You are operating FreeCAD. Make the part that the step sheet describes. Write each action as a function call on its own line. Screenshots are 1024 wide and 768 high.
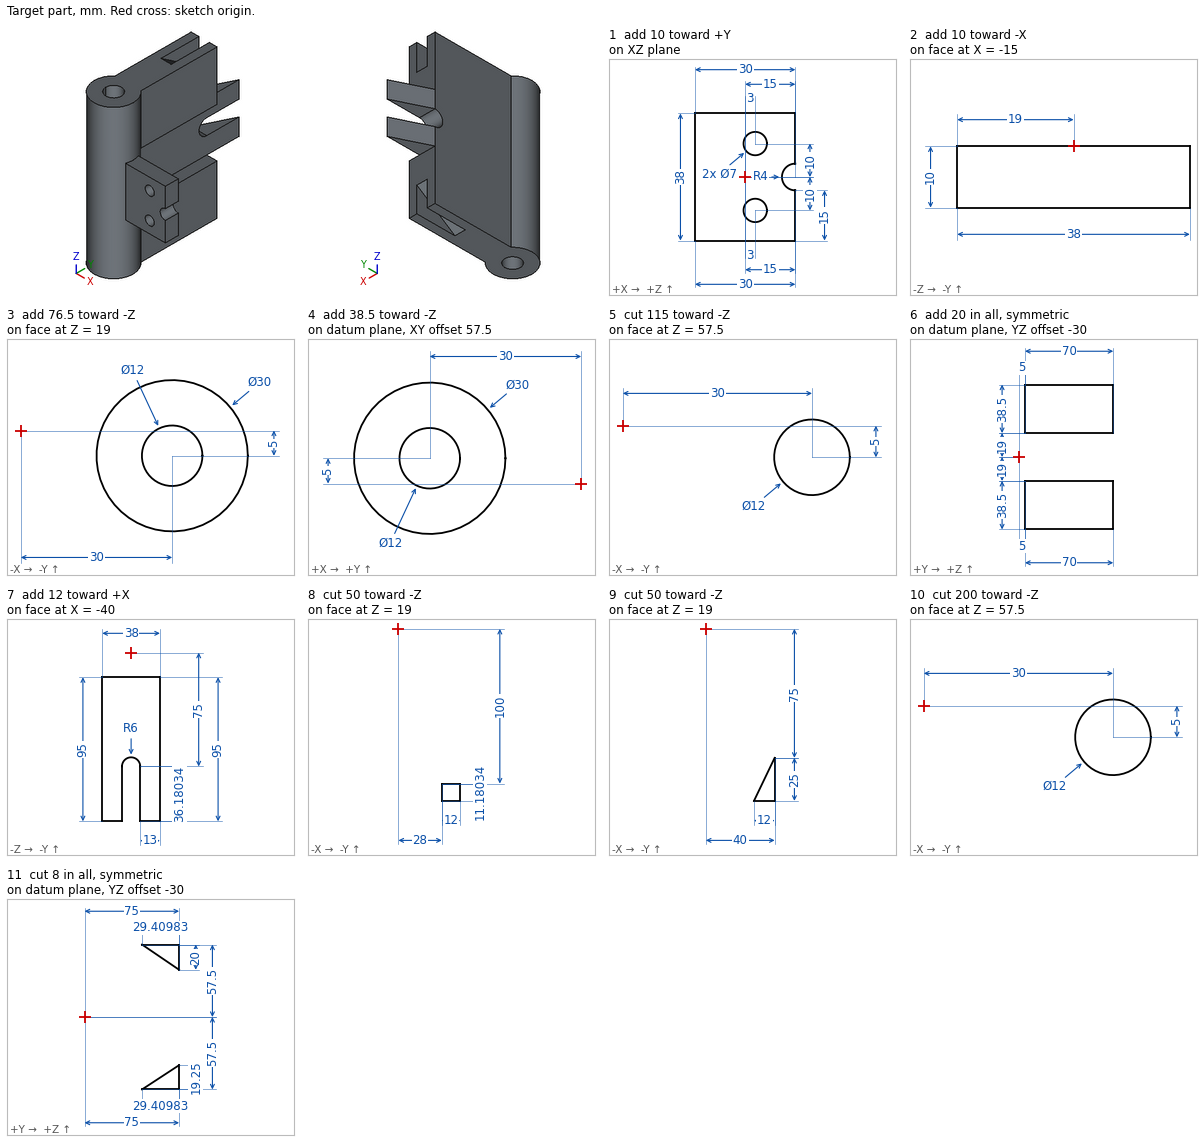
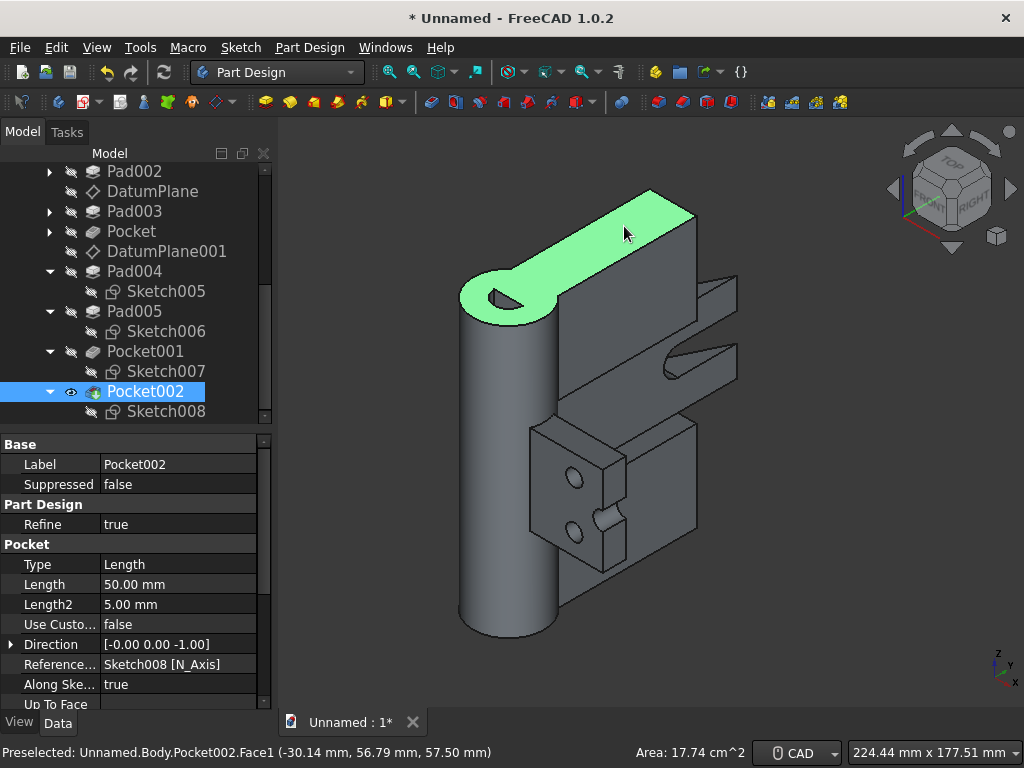
click(84, 102)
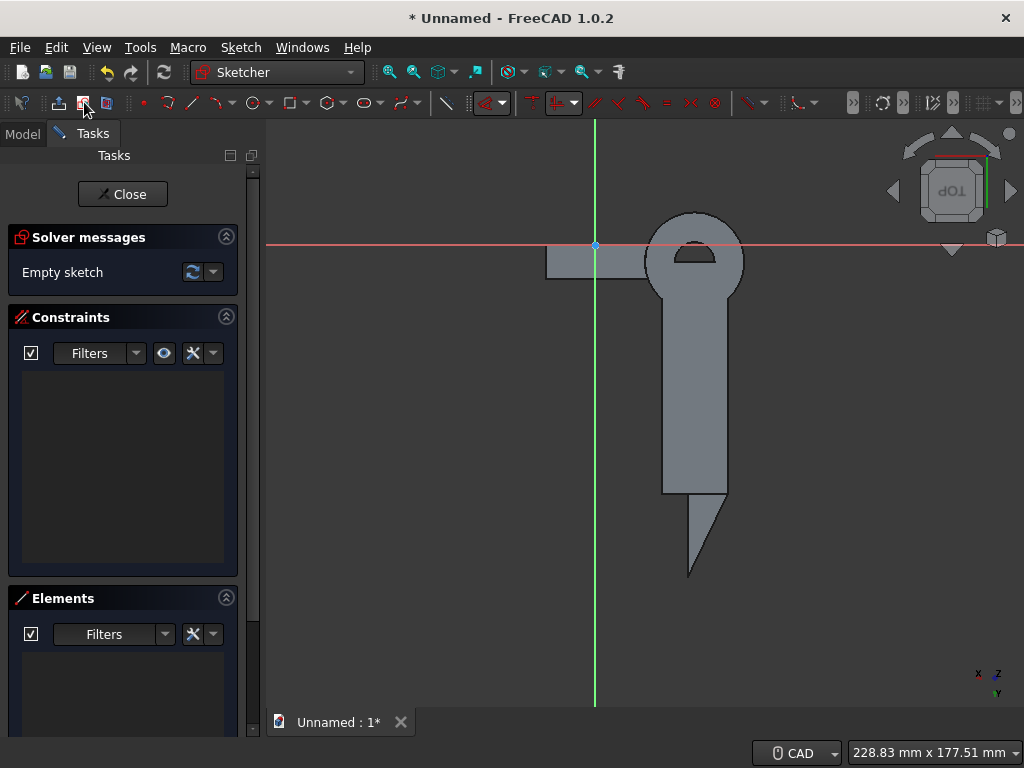
scroll(709, 243, up, 11)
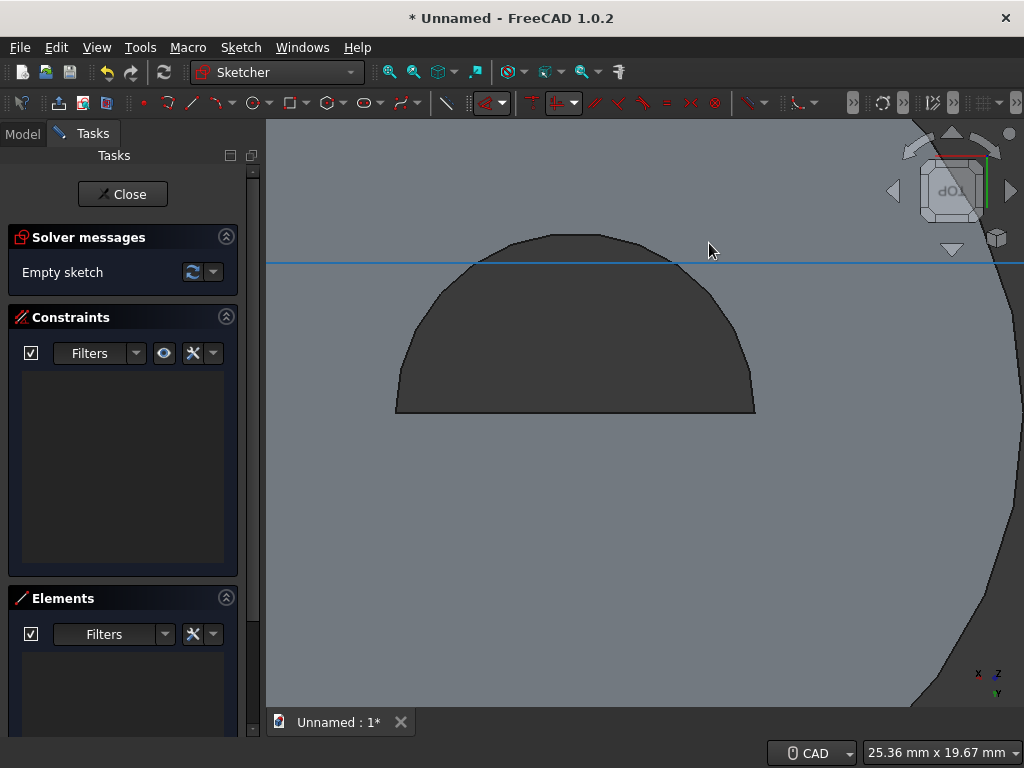
click(254, 104)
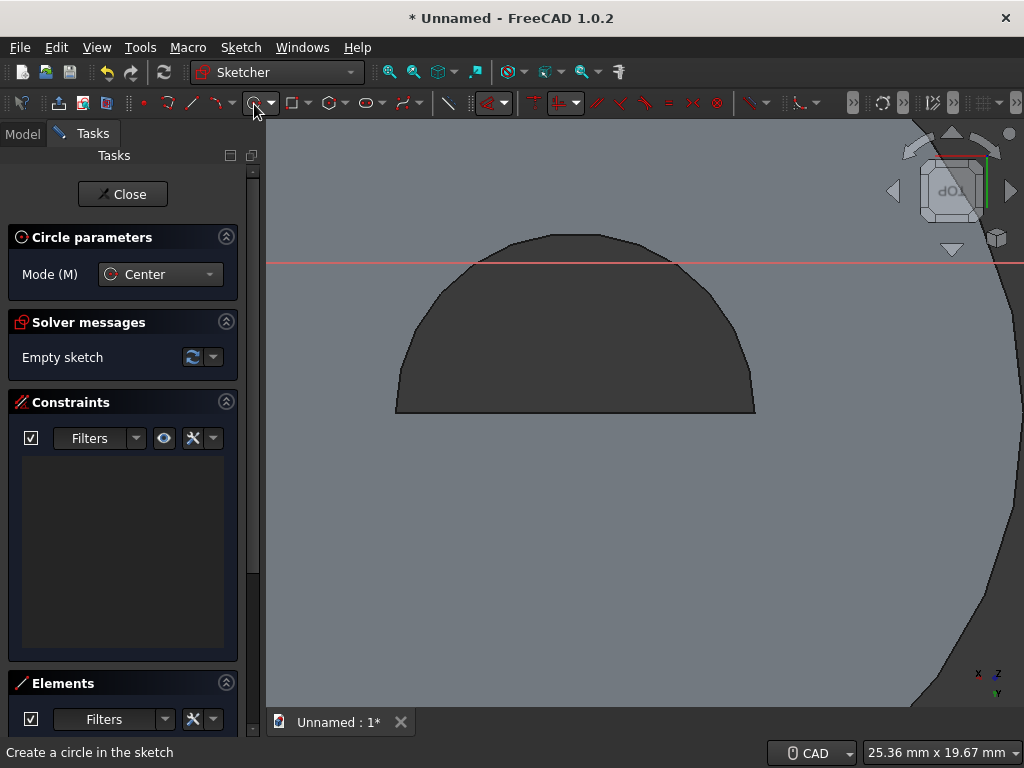
click(575, 413)
click(702, 286)
key(Escape)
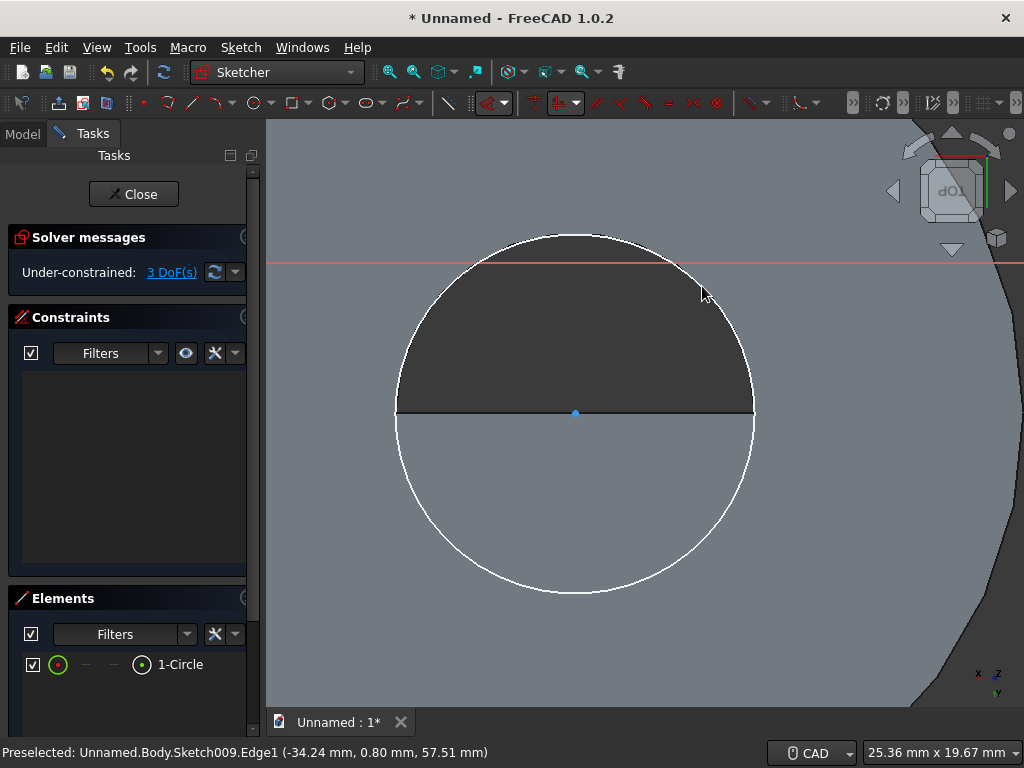
click(702, 287)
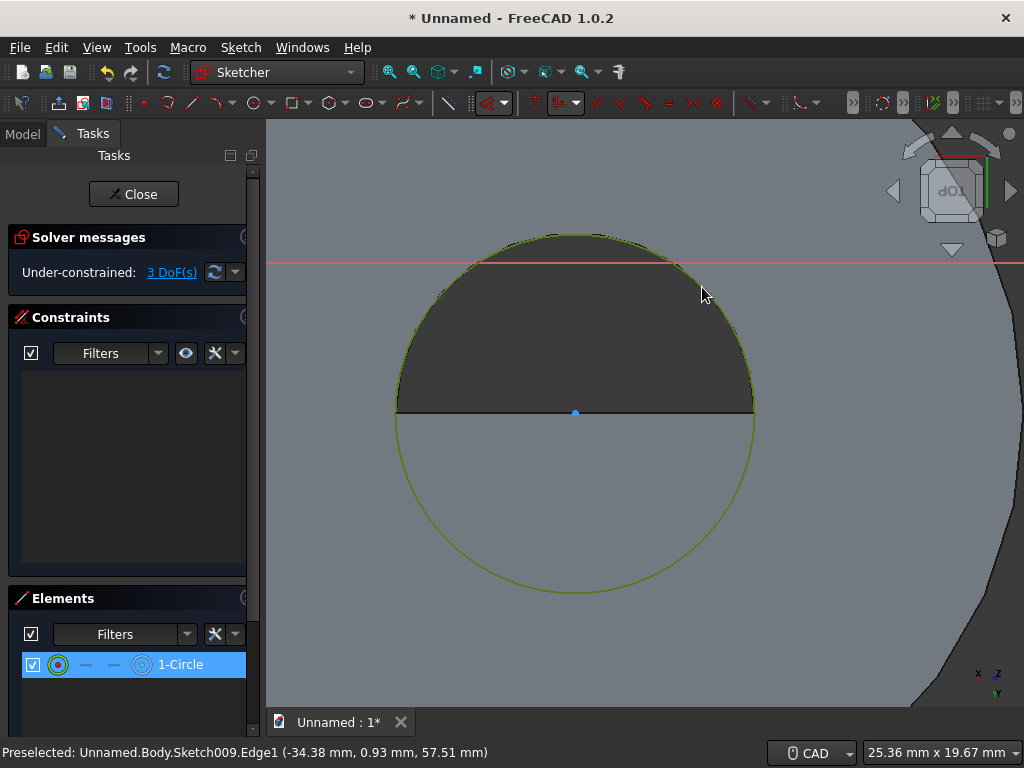
click(506, 104)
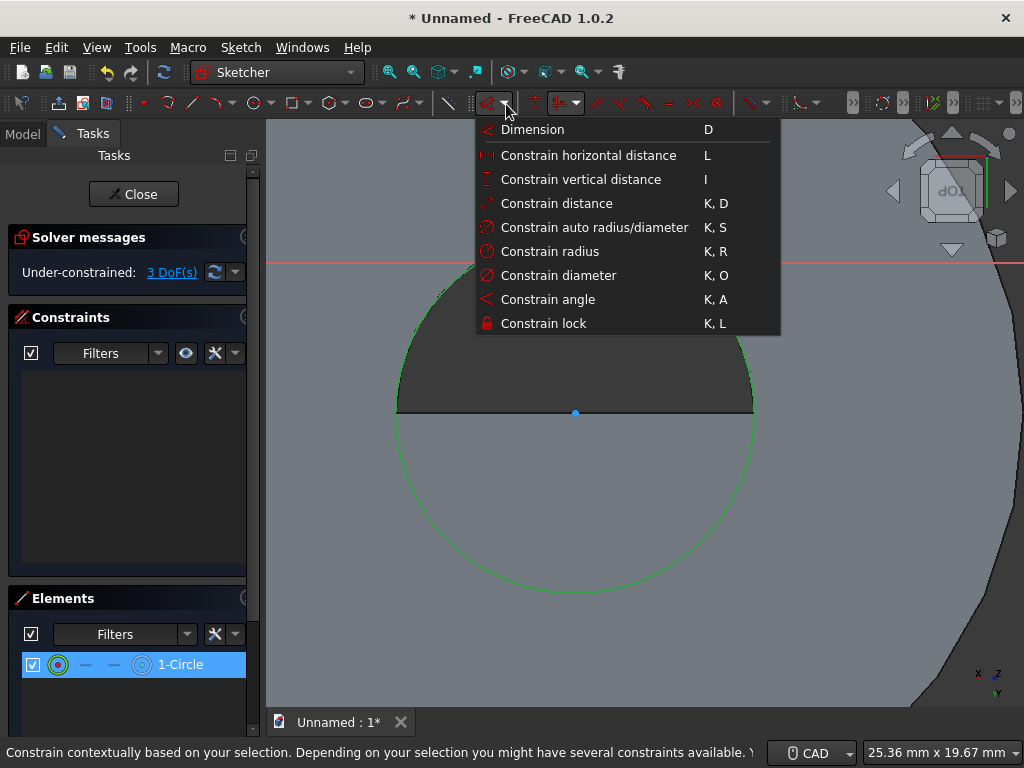
click(628, 275)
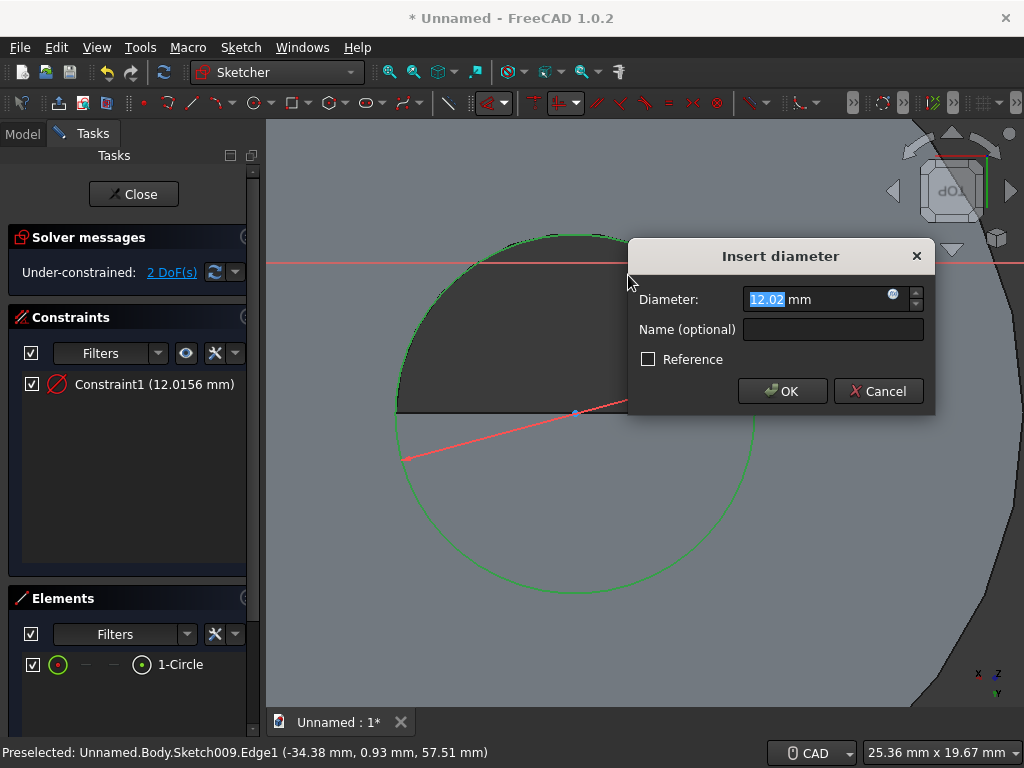
text(12)
key(Return)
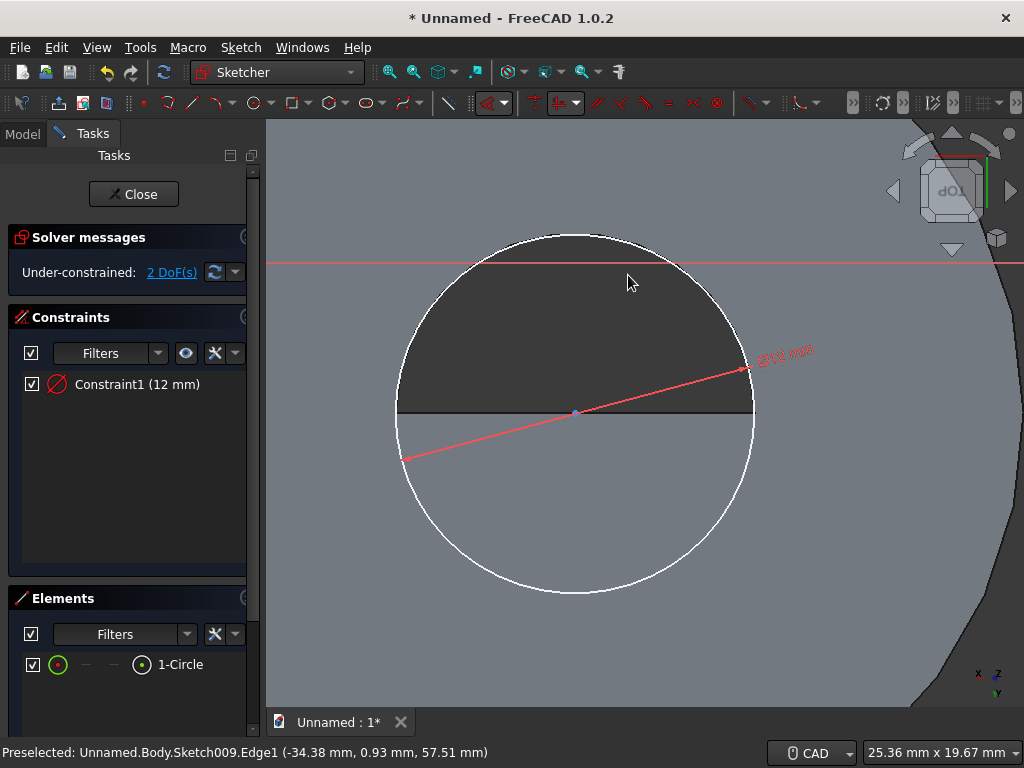
click(575, 414)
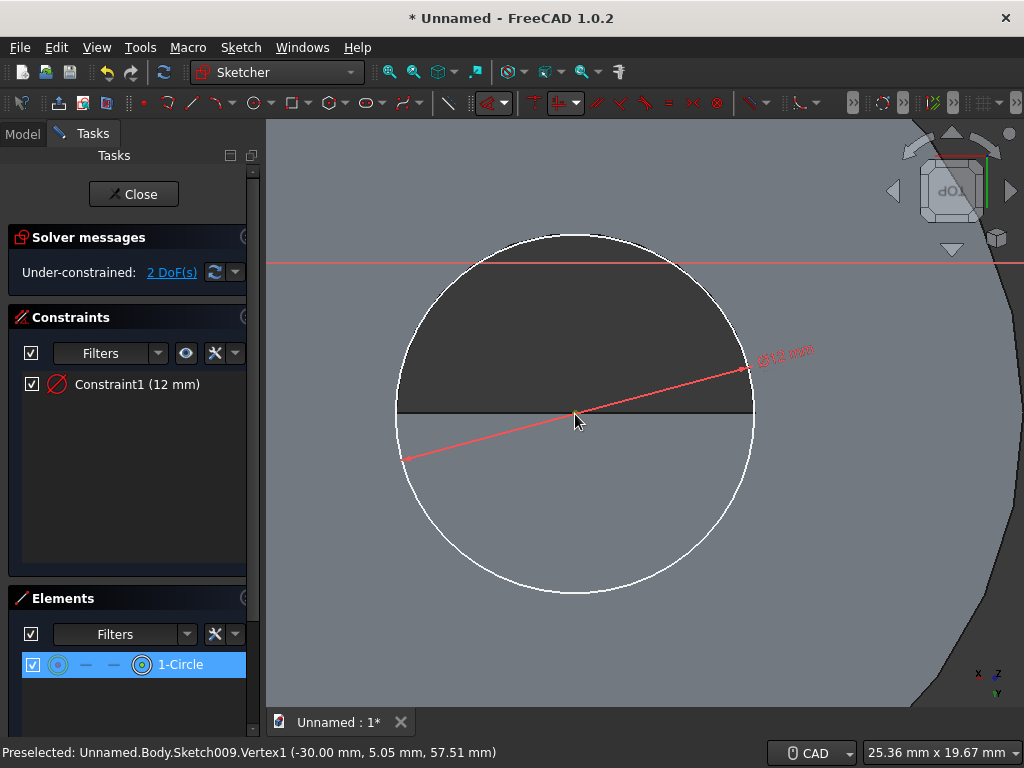
key(i)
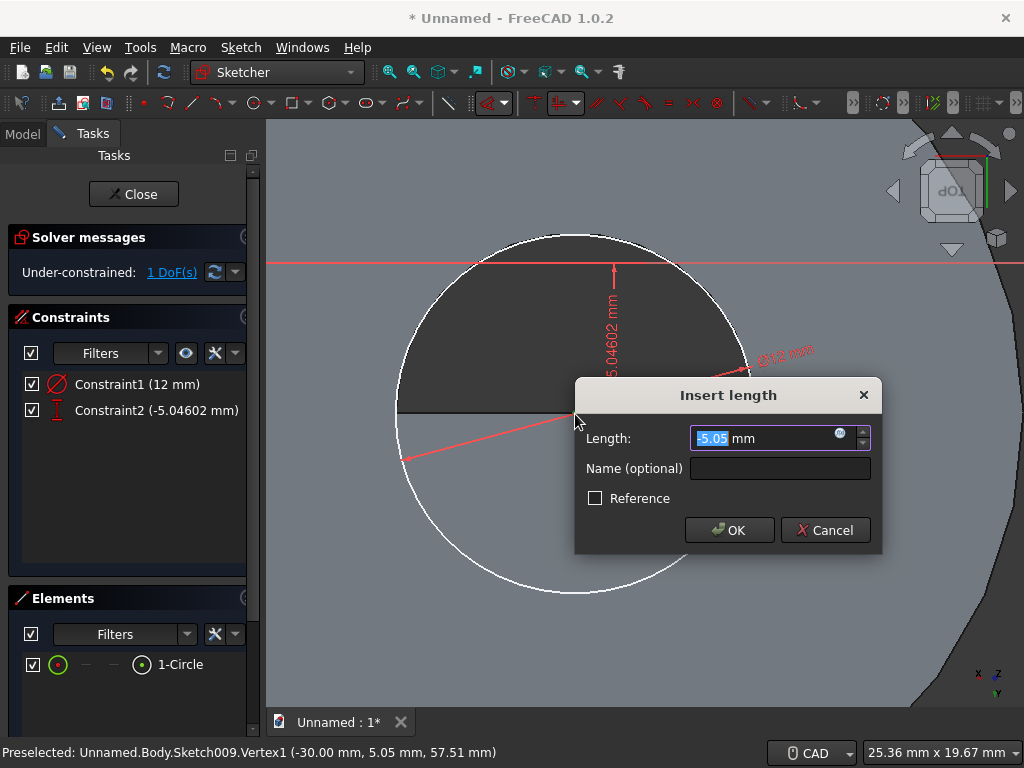
text(-5)
key(Return)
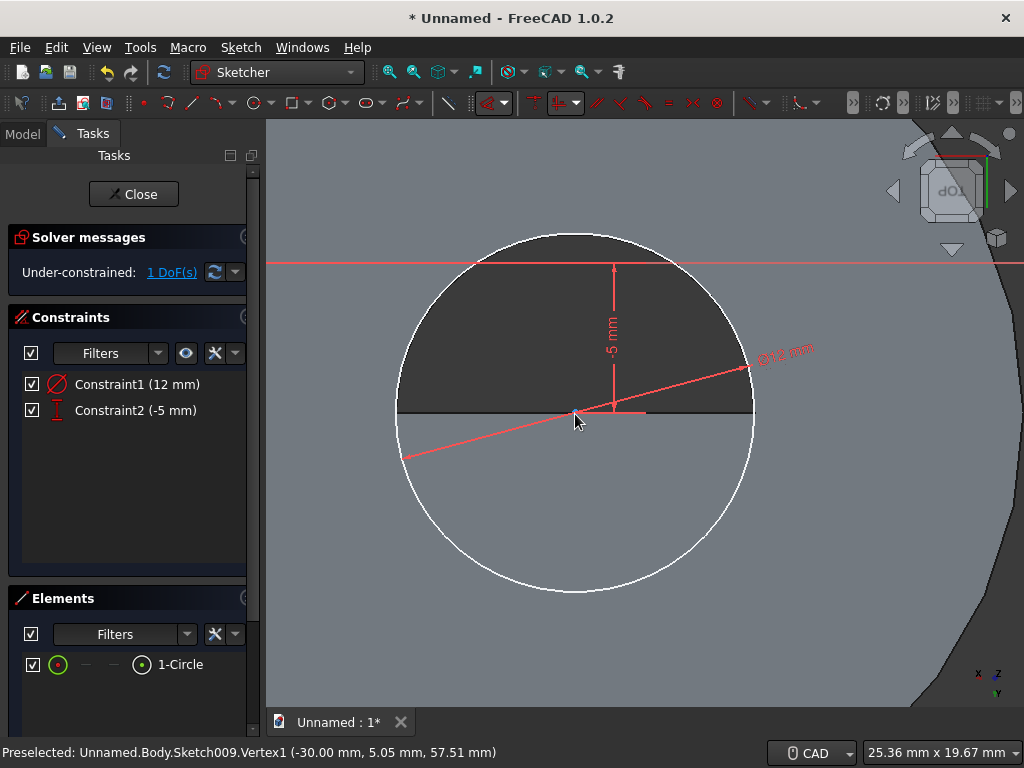
click(575, 413)